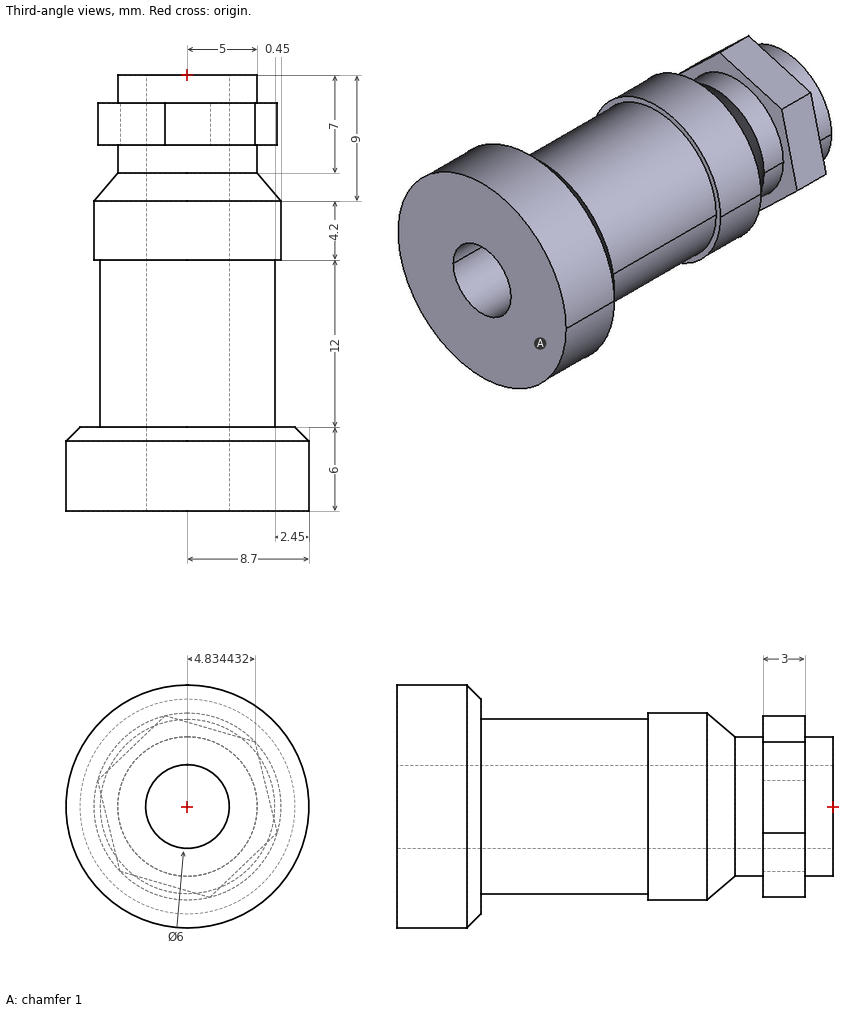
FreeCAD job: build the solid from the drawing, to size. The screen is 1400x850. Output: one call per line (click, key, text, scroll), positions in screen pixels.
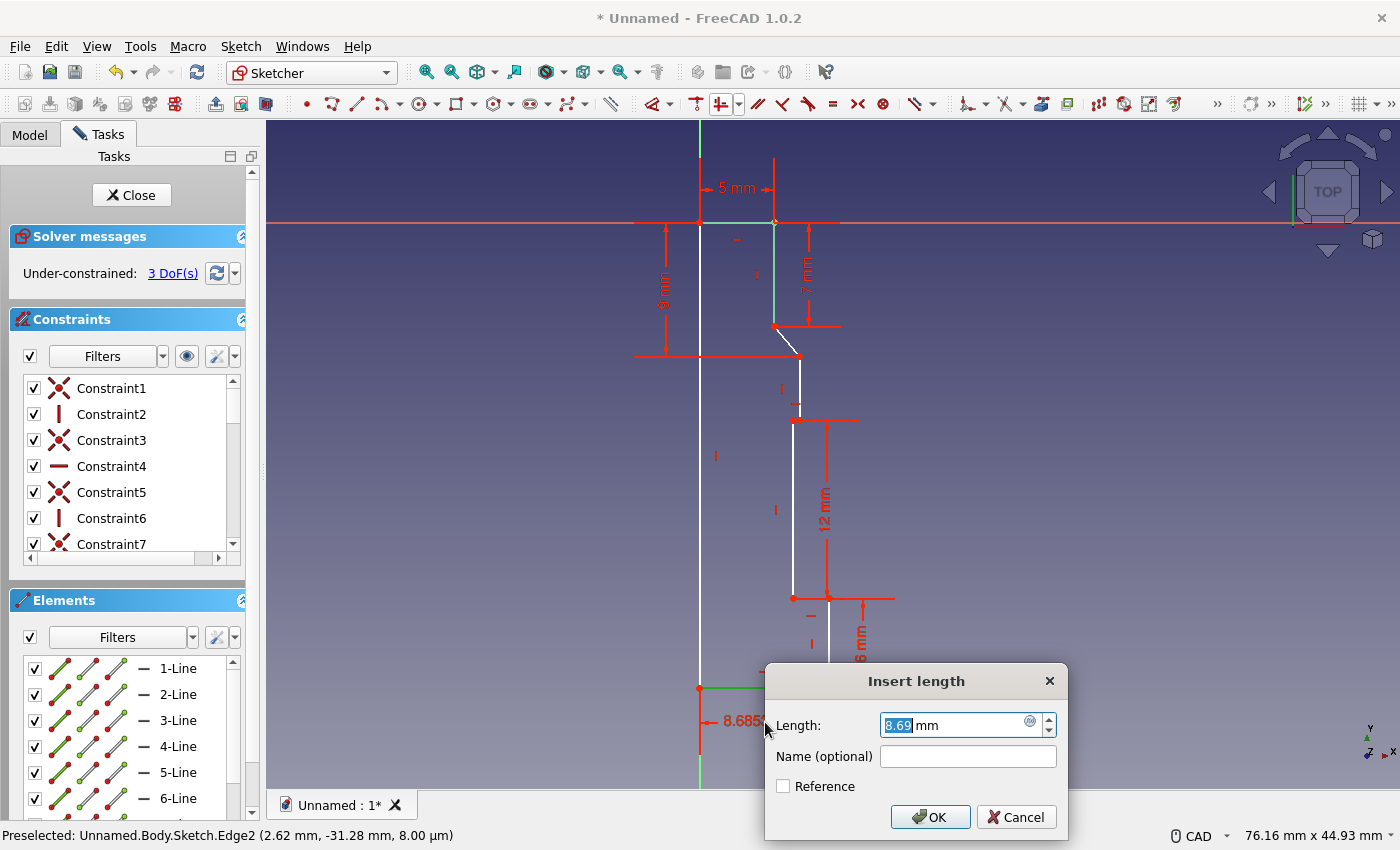
text(8.7)
key(Return)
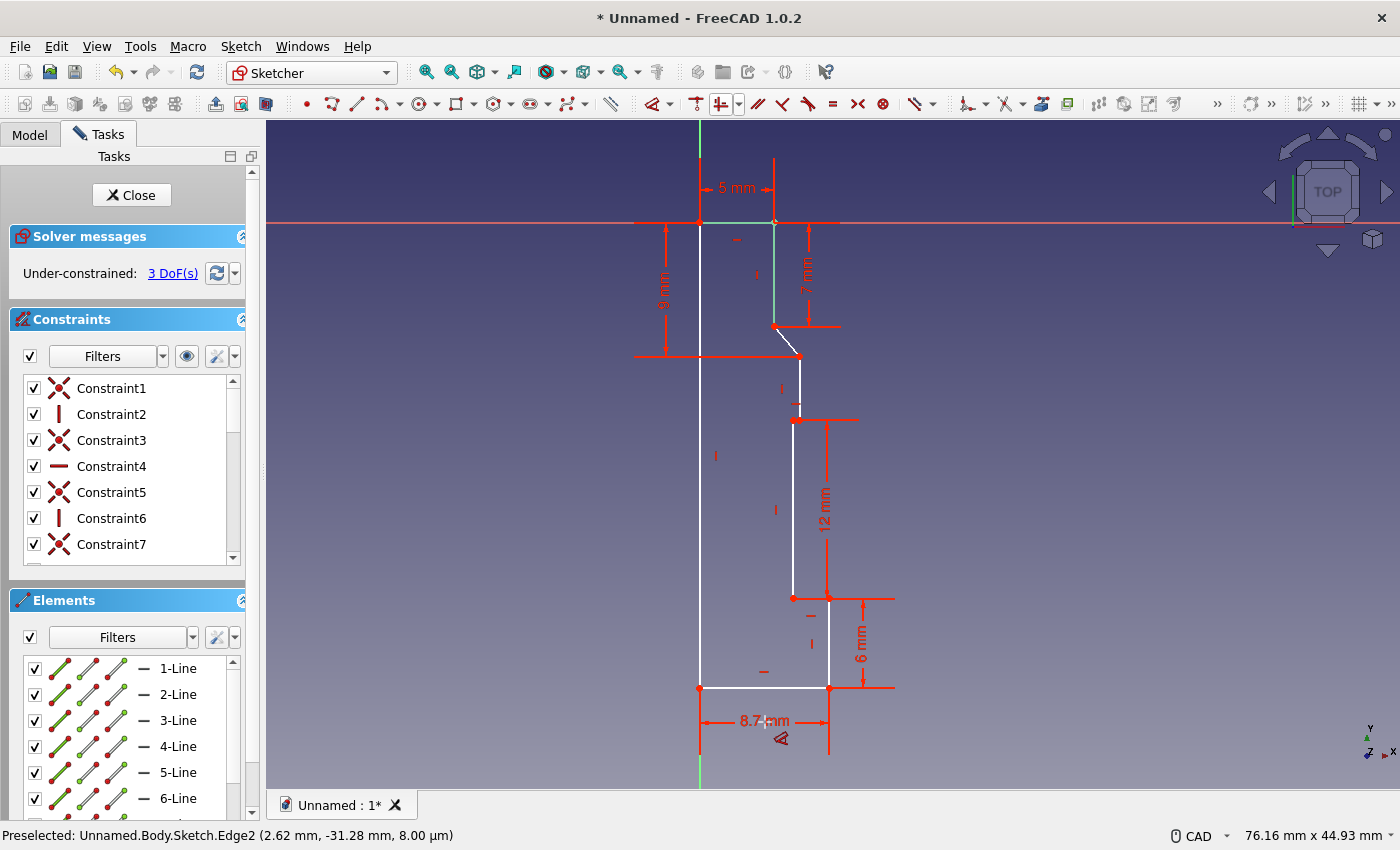
click(800, 401)
click(834, 388)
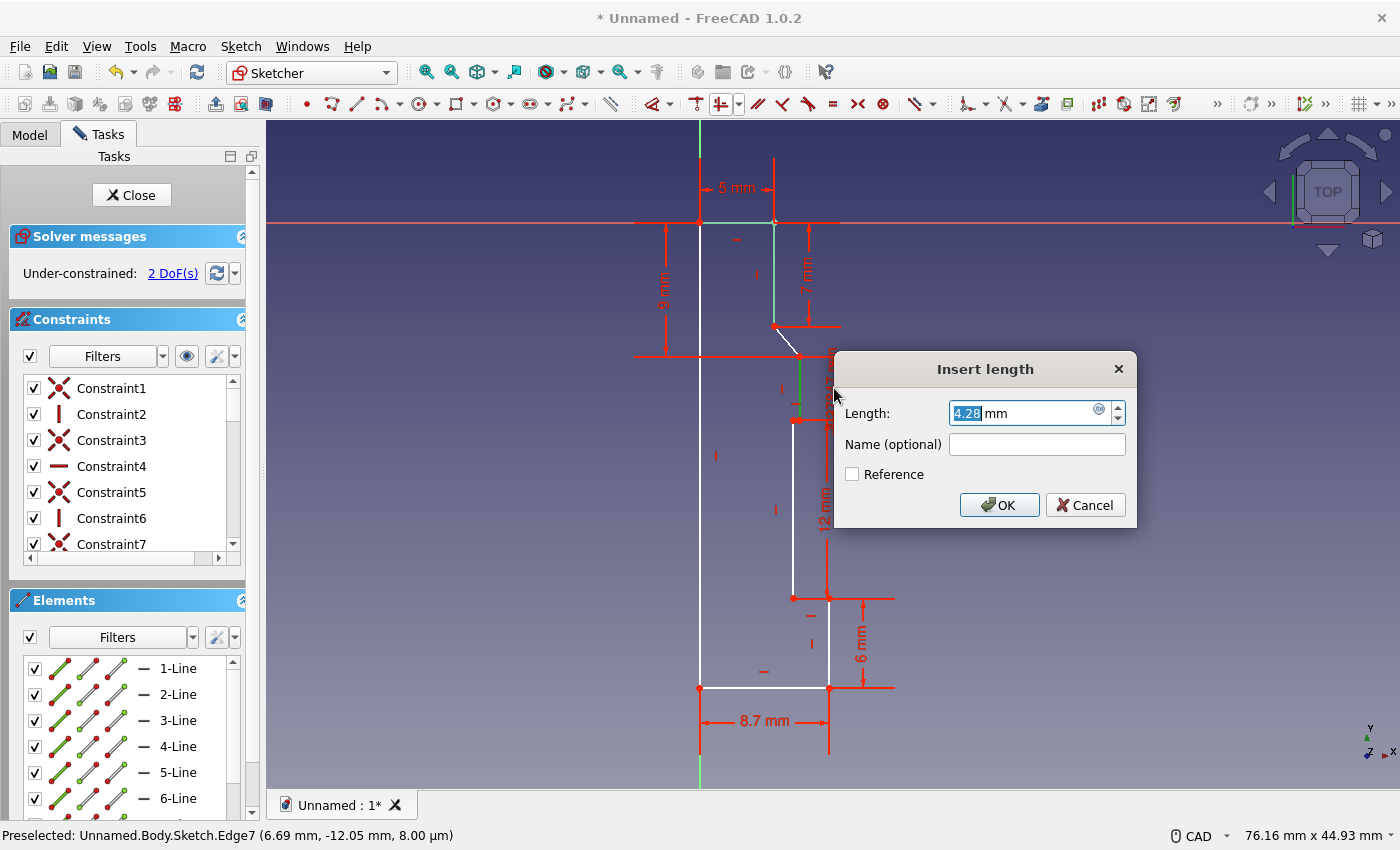
text(4.2)
key(Return)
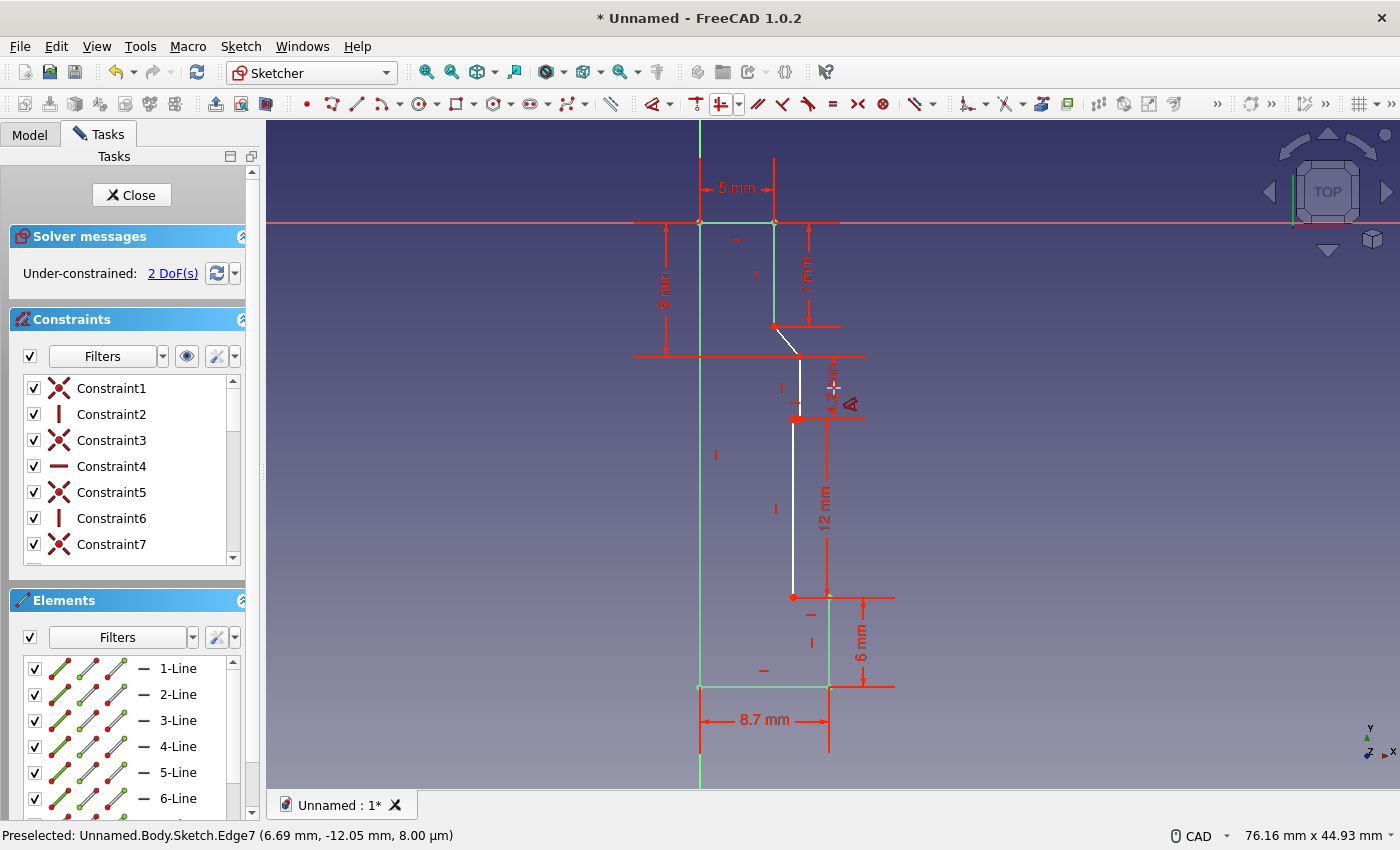
scroll(819, 598, up, 2)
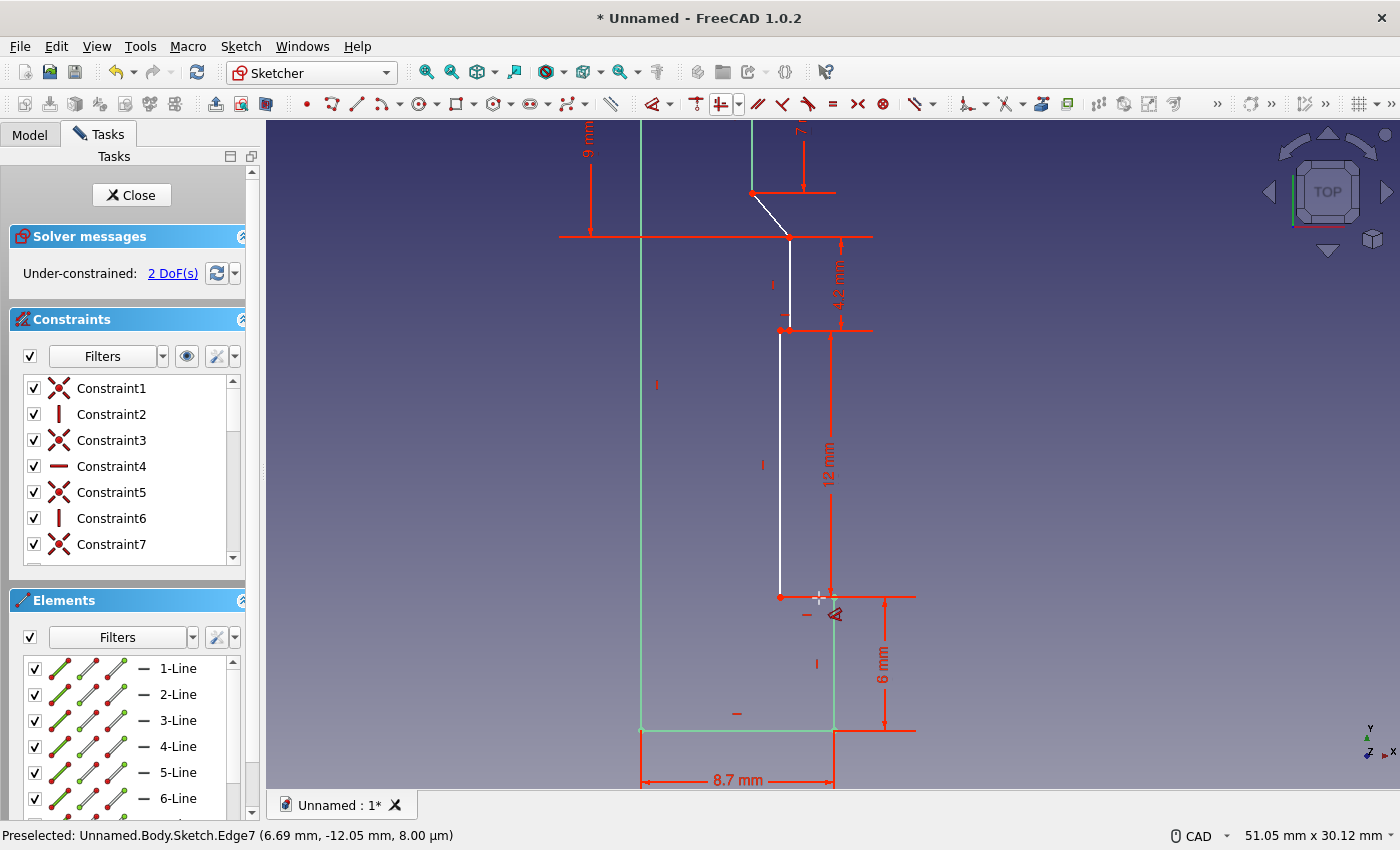
click(818, 597)
click(807, 631)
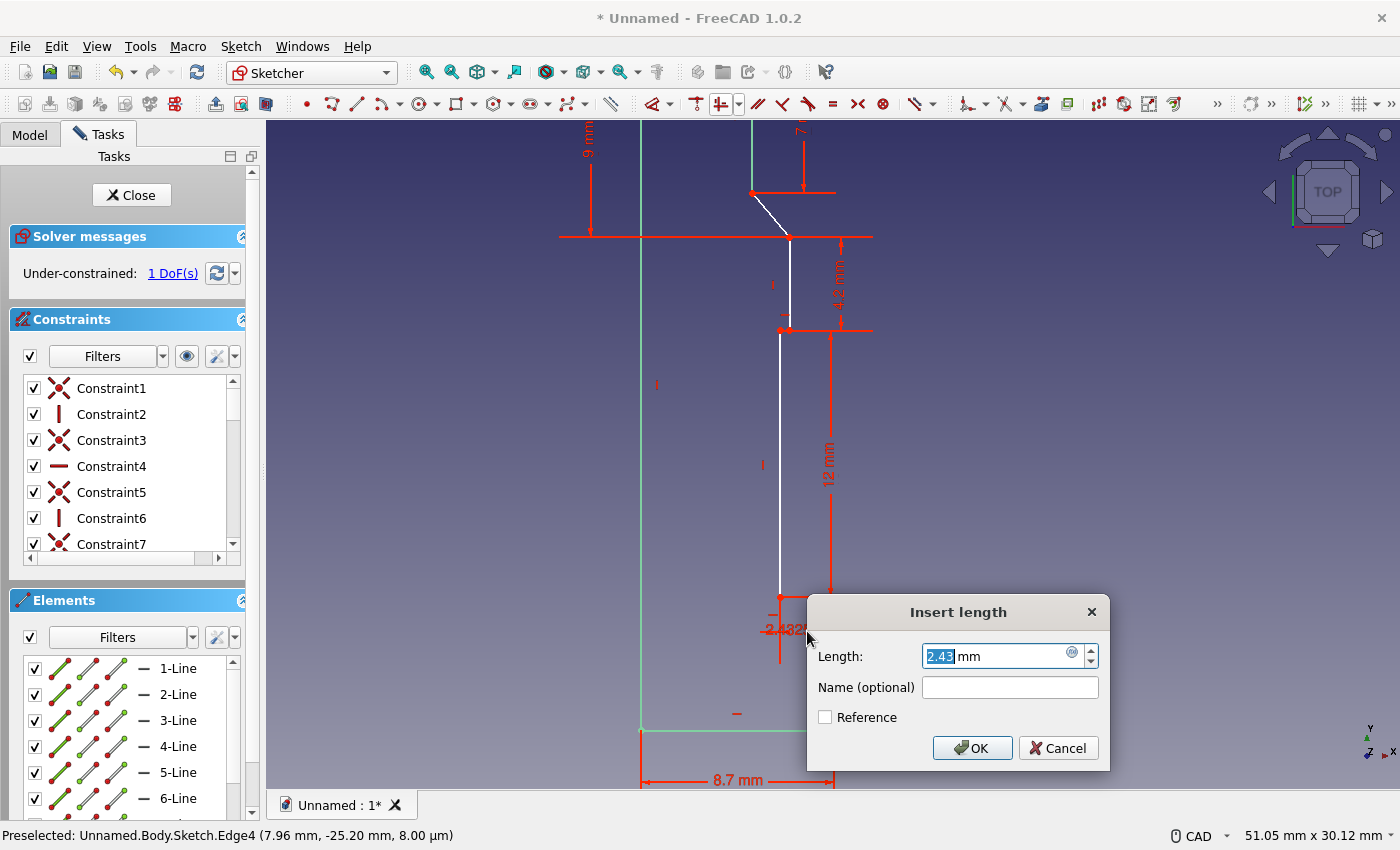
text(2.45)
key(Return)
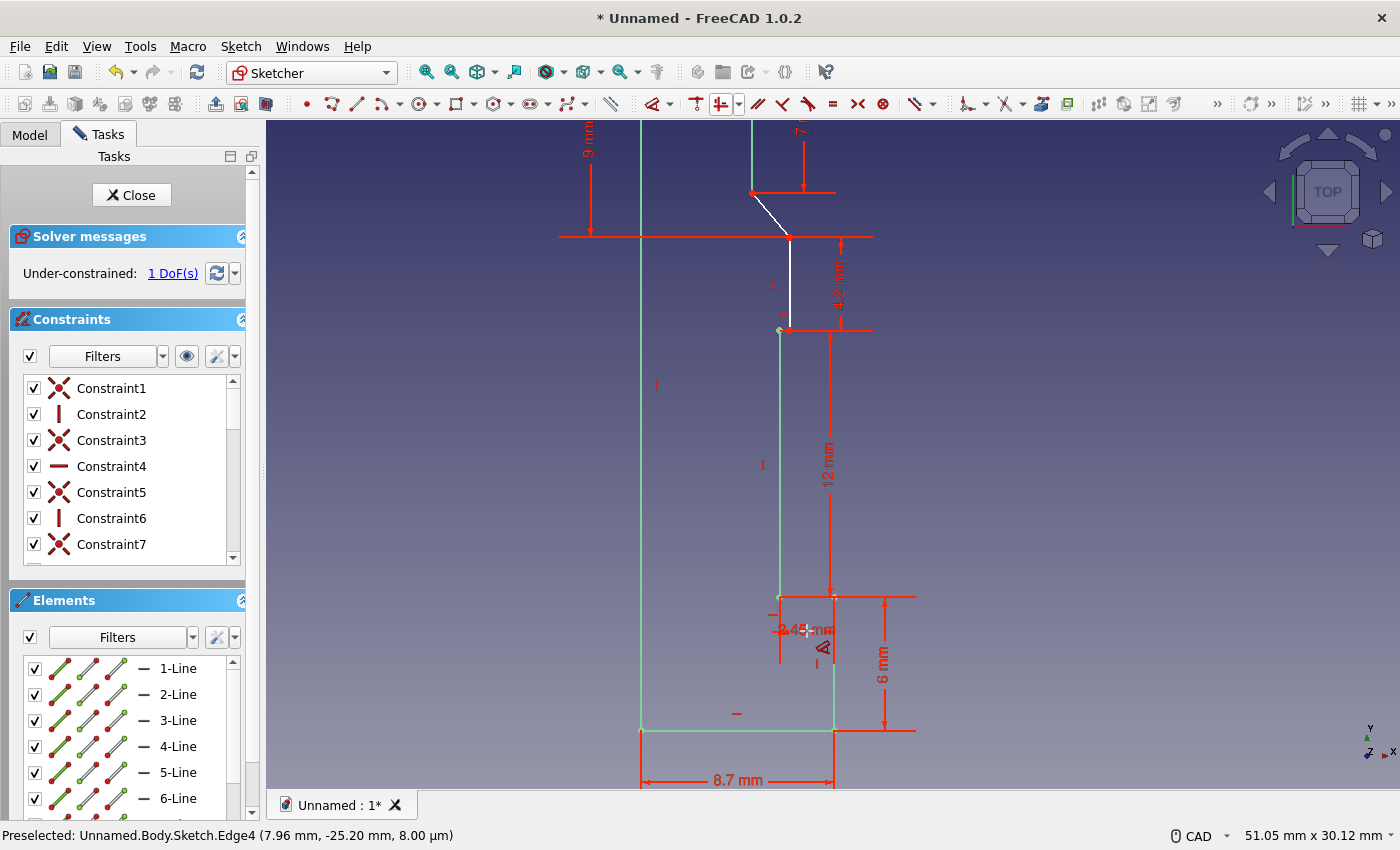
scroll(785, 331, up, 7)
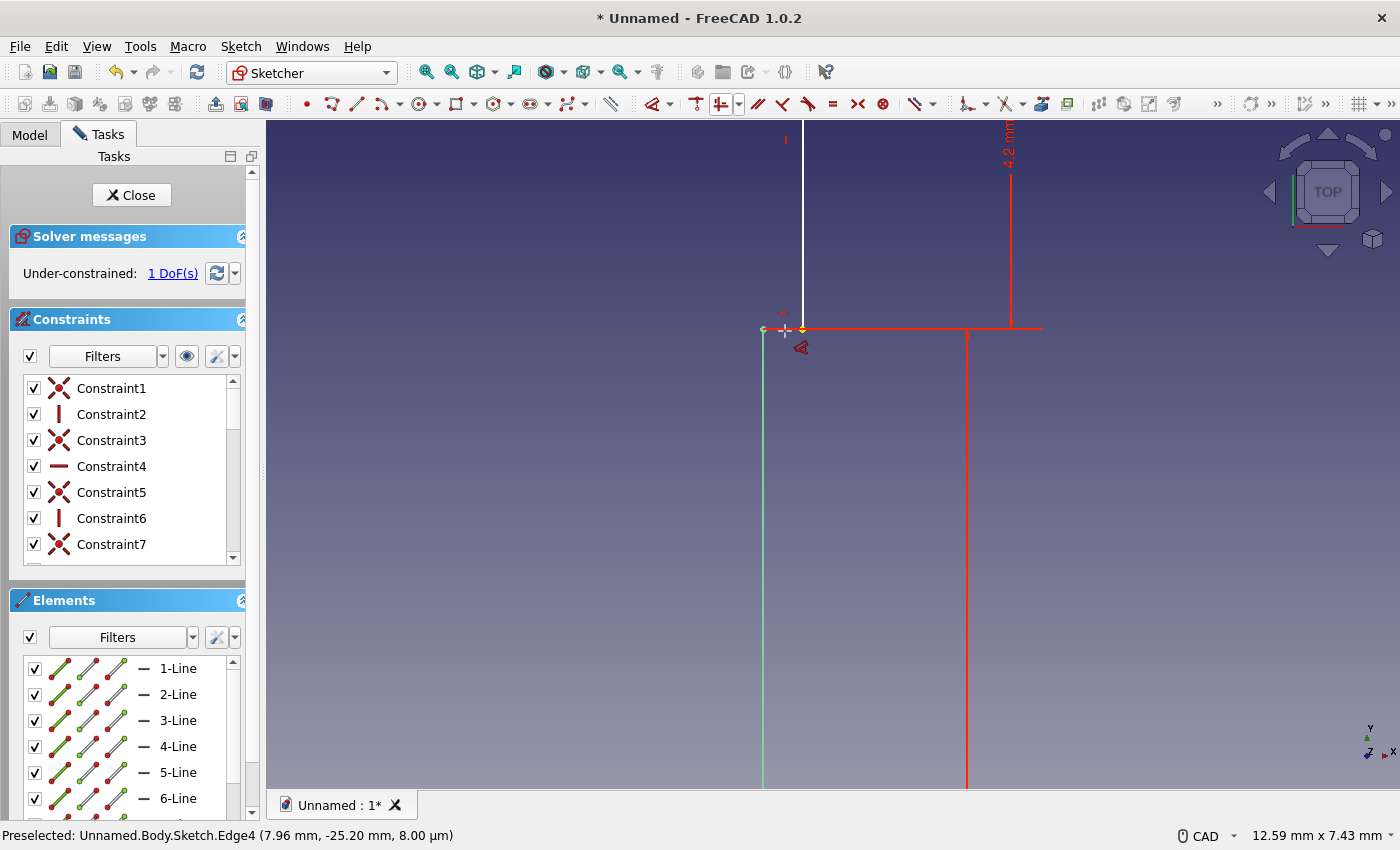
click(783, 329)
click(783, 295)